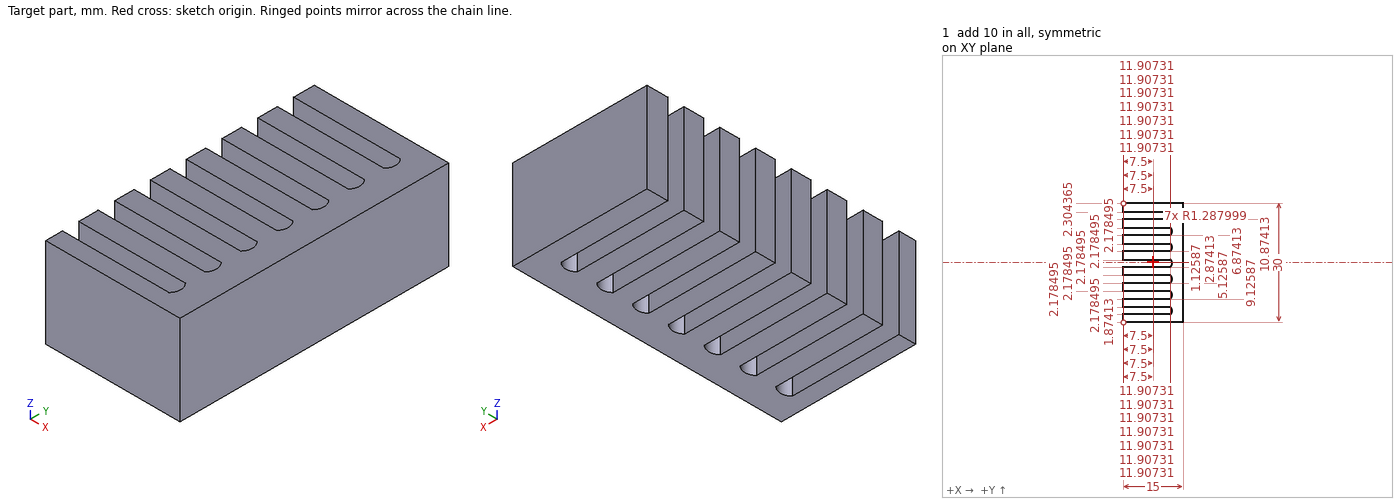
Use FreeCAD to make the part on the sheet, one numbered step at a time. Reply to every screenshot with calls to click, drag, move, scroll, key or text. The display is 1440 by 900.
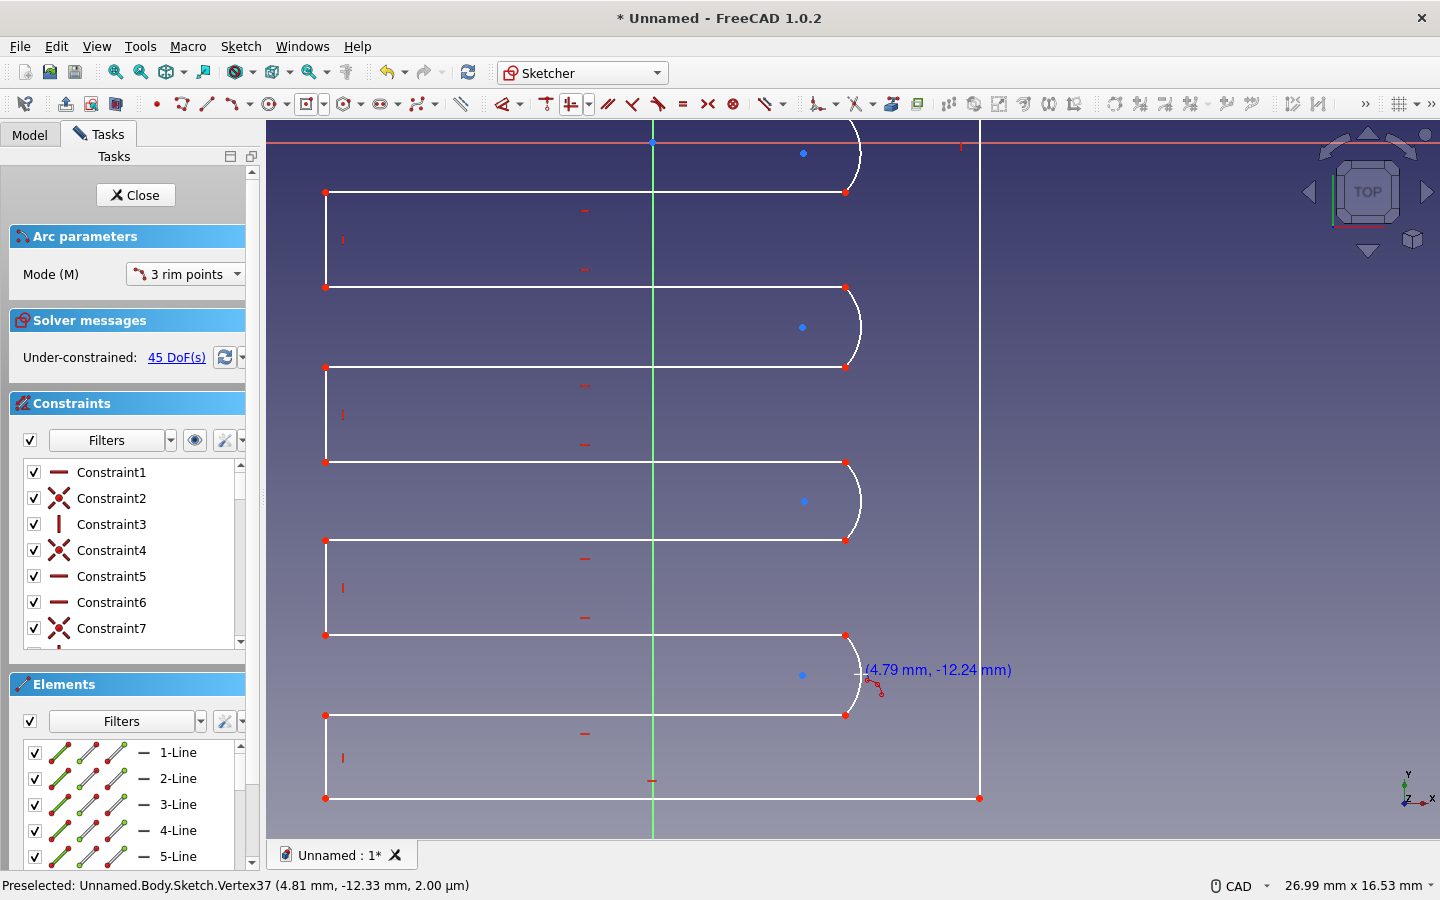
scroll(861, 676, down, 5)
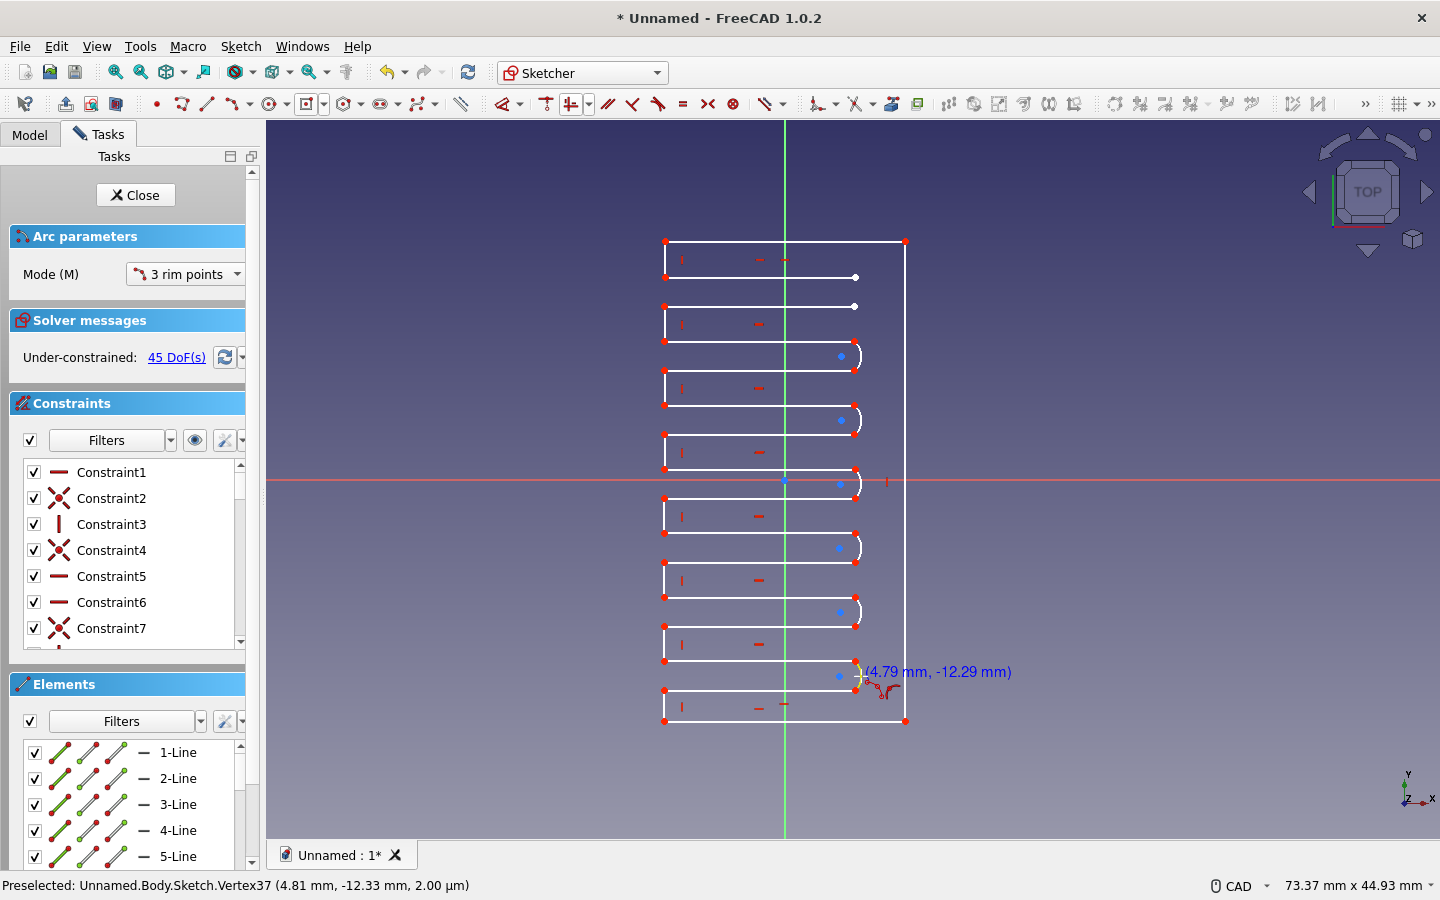
click(855, 278)
click(855, 307)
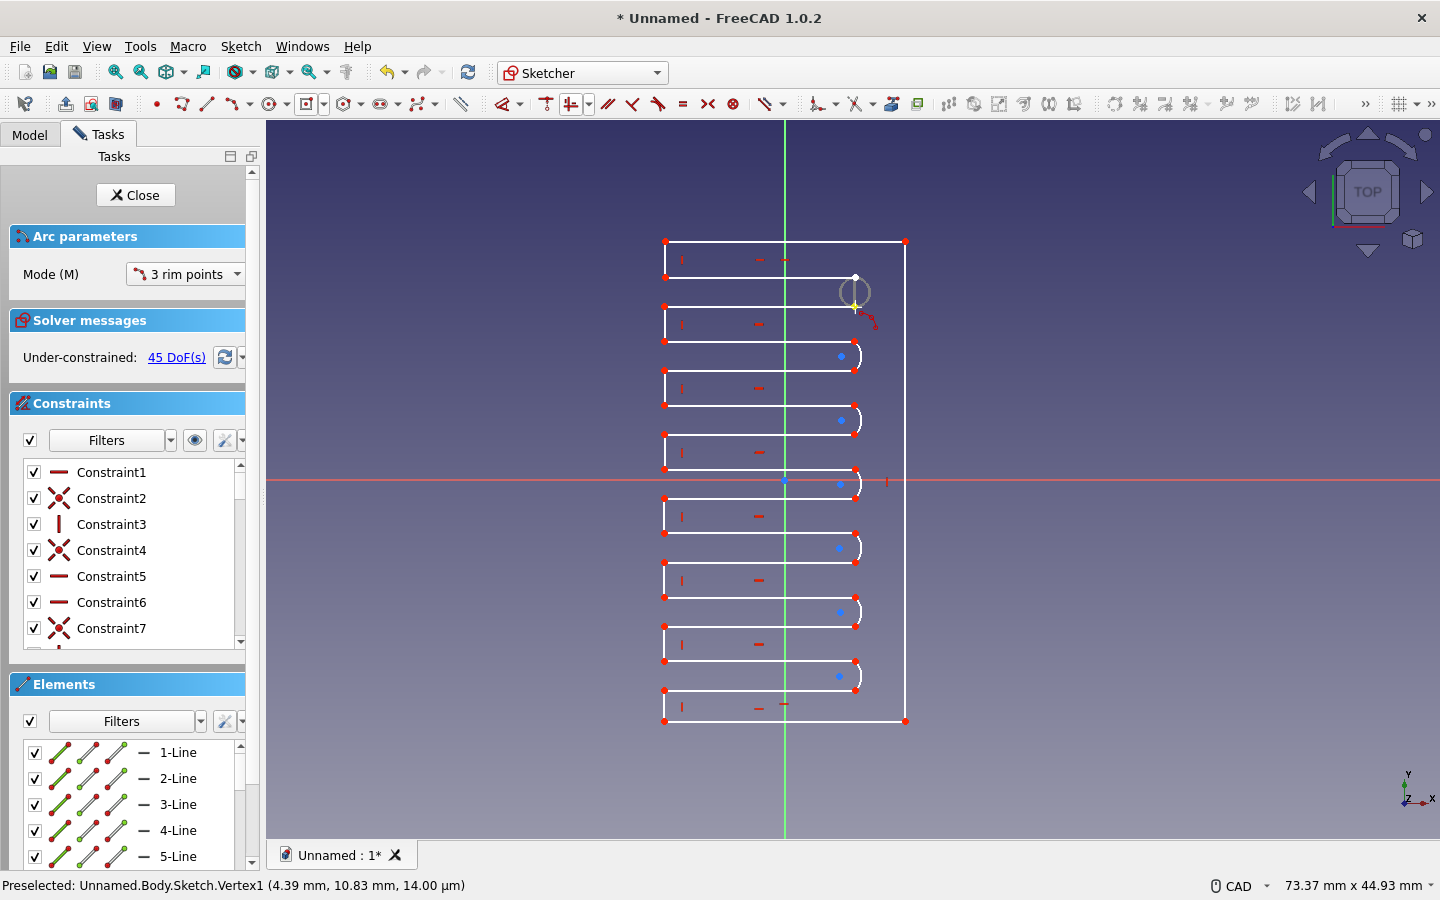
scroll(861, 292, up, 5)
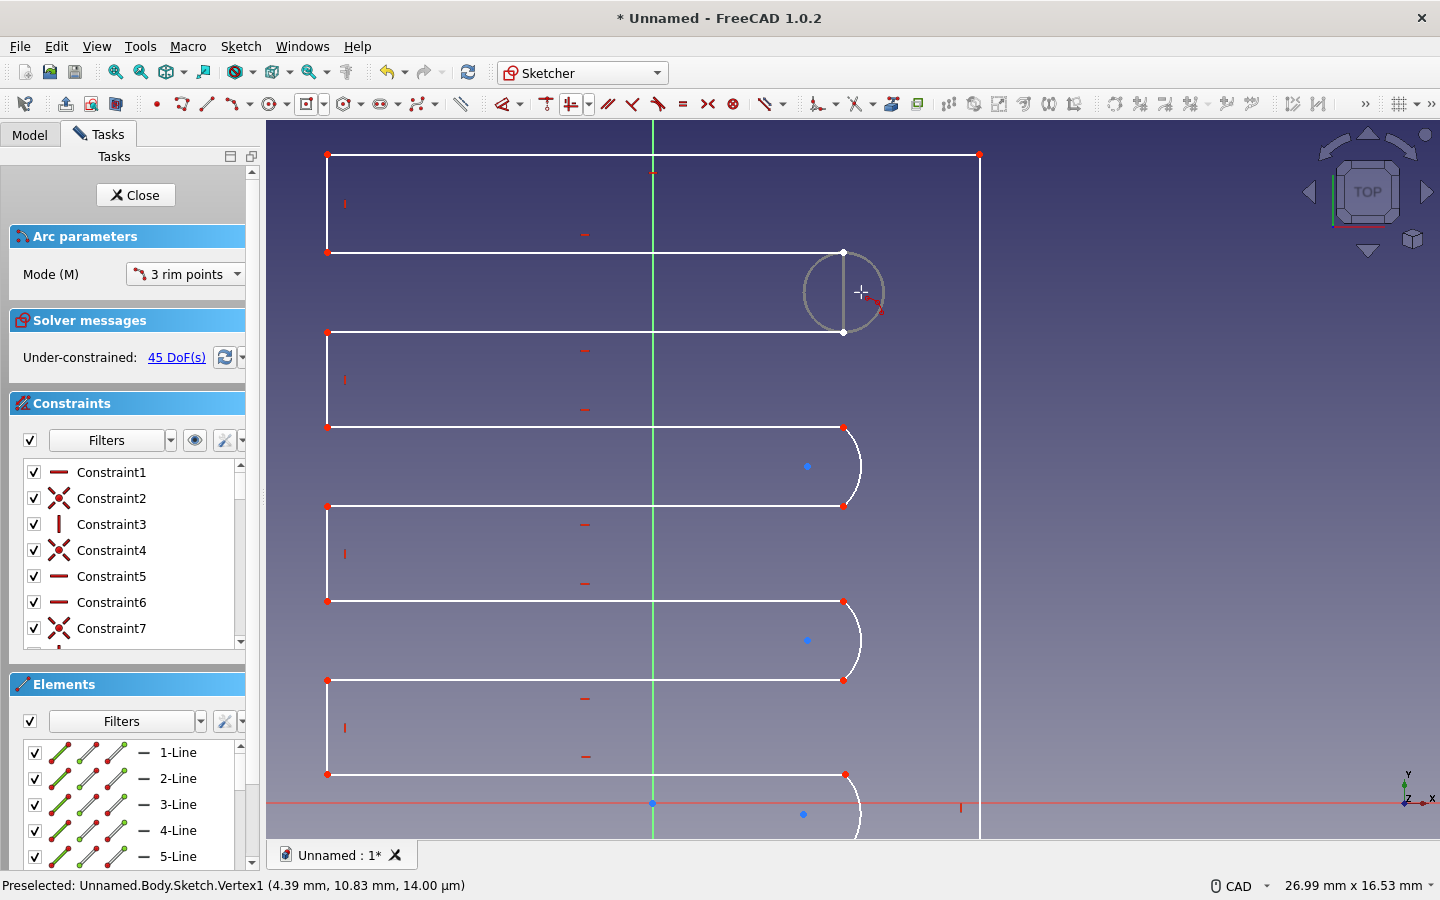
click(861, 291)
key(Escape)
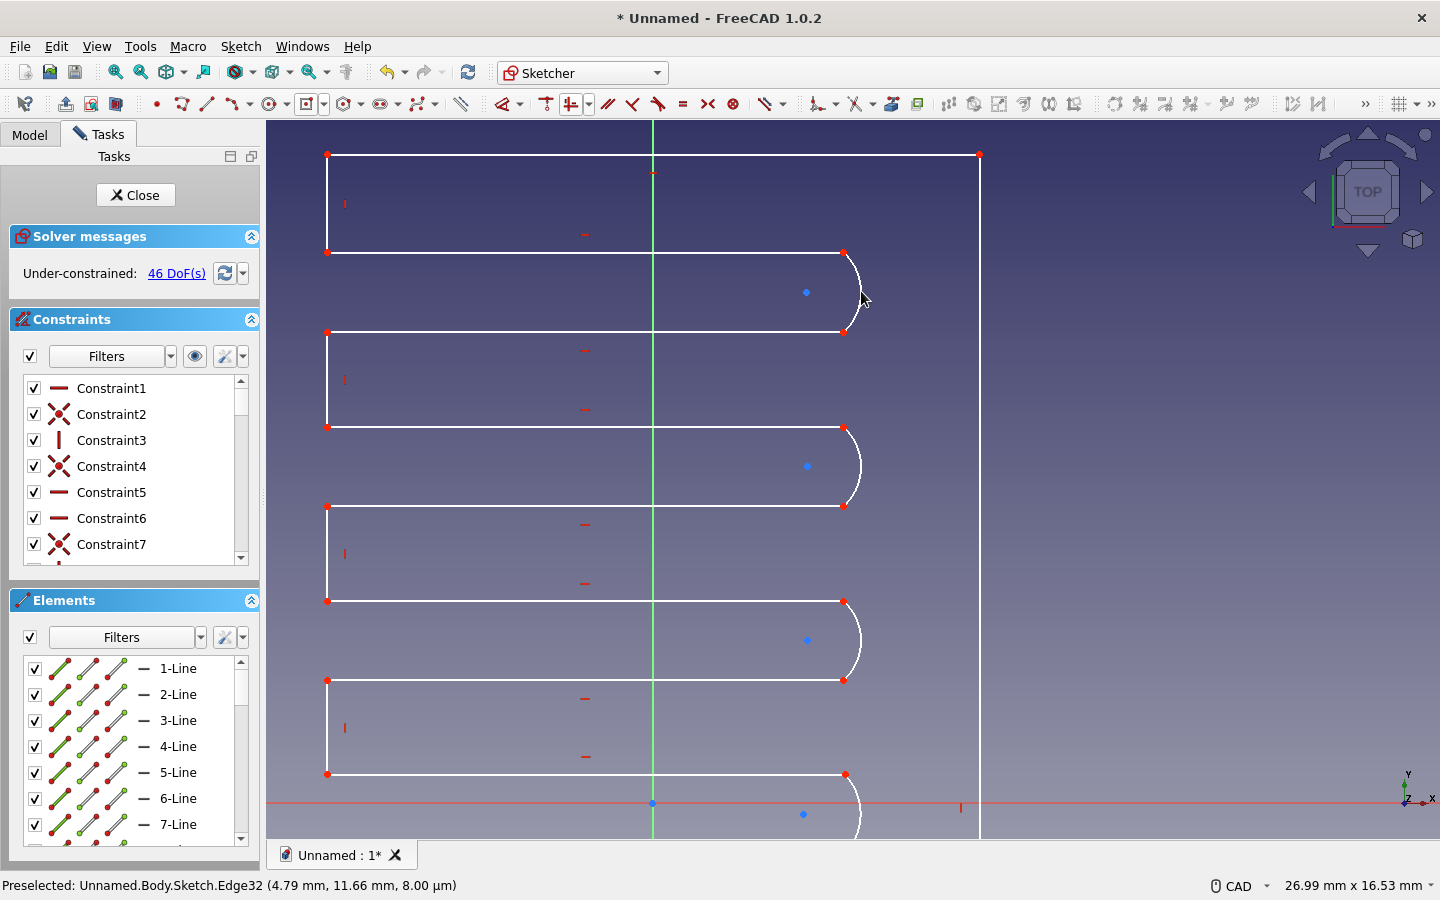
click(858, 484)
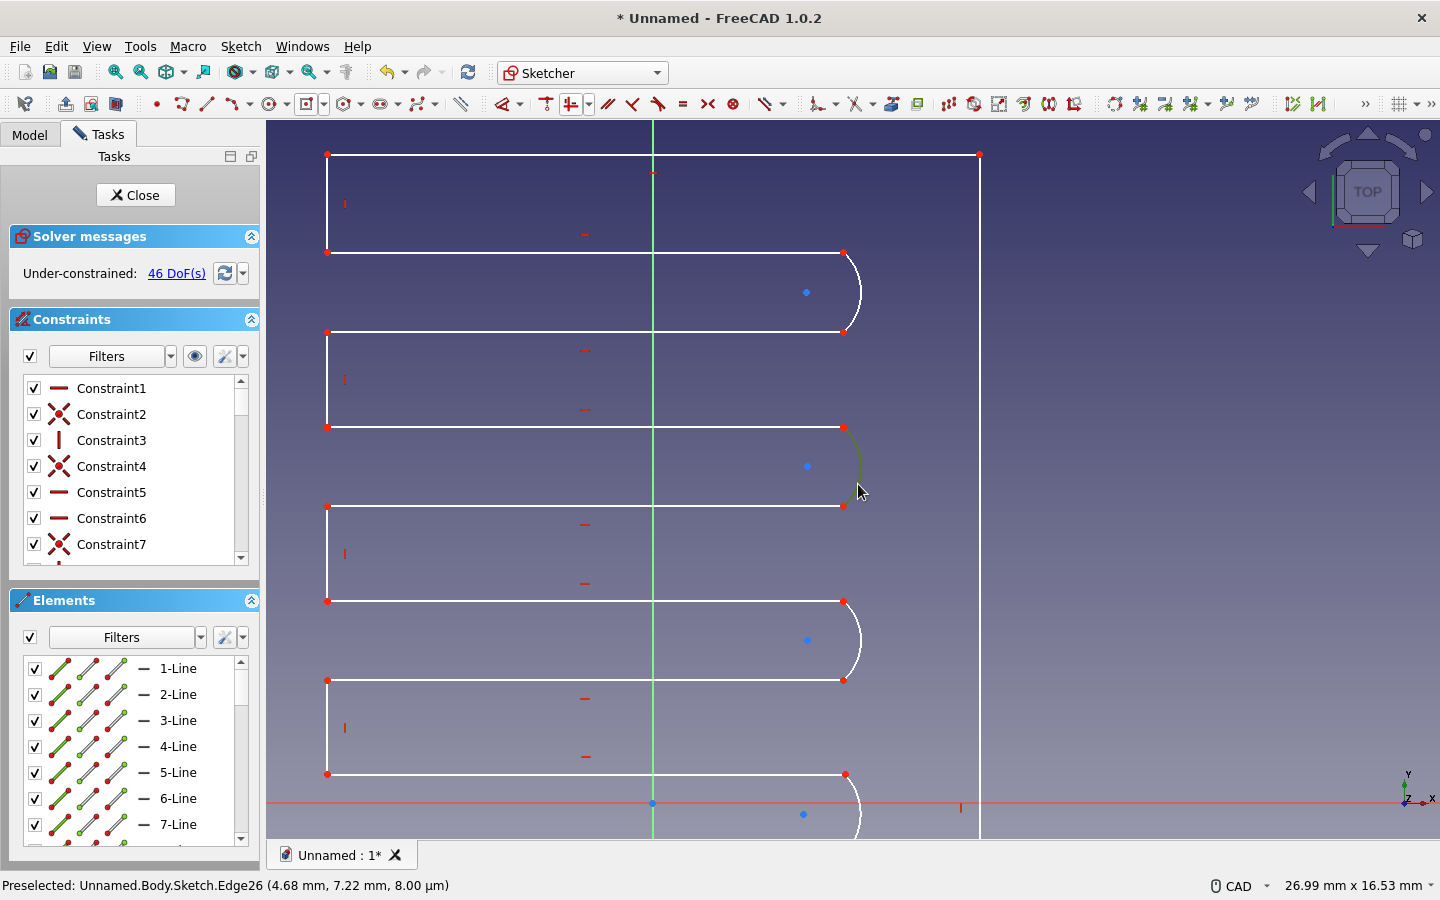
click(858, 658)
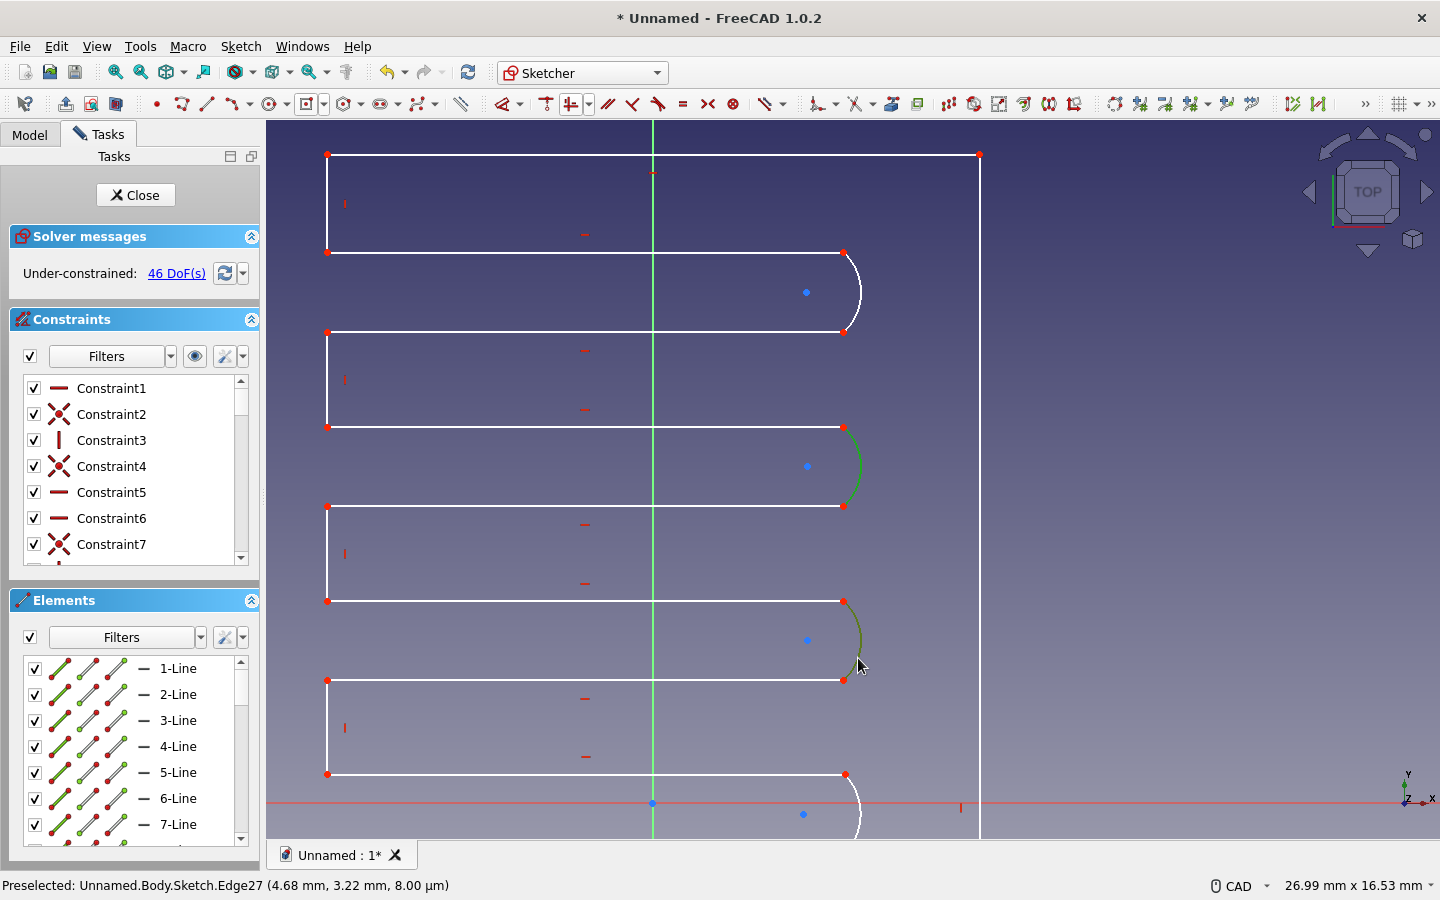
click(855, 789)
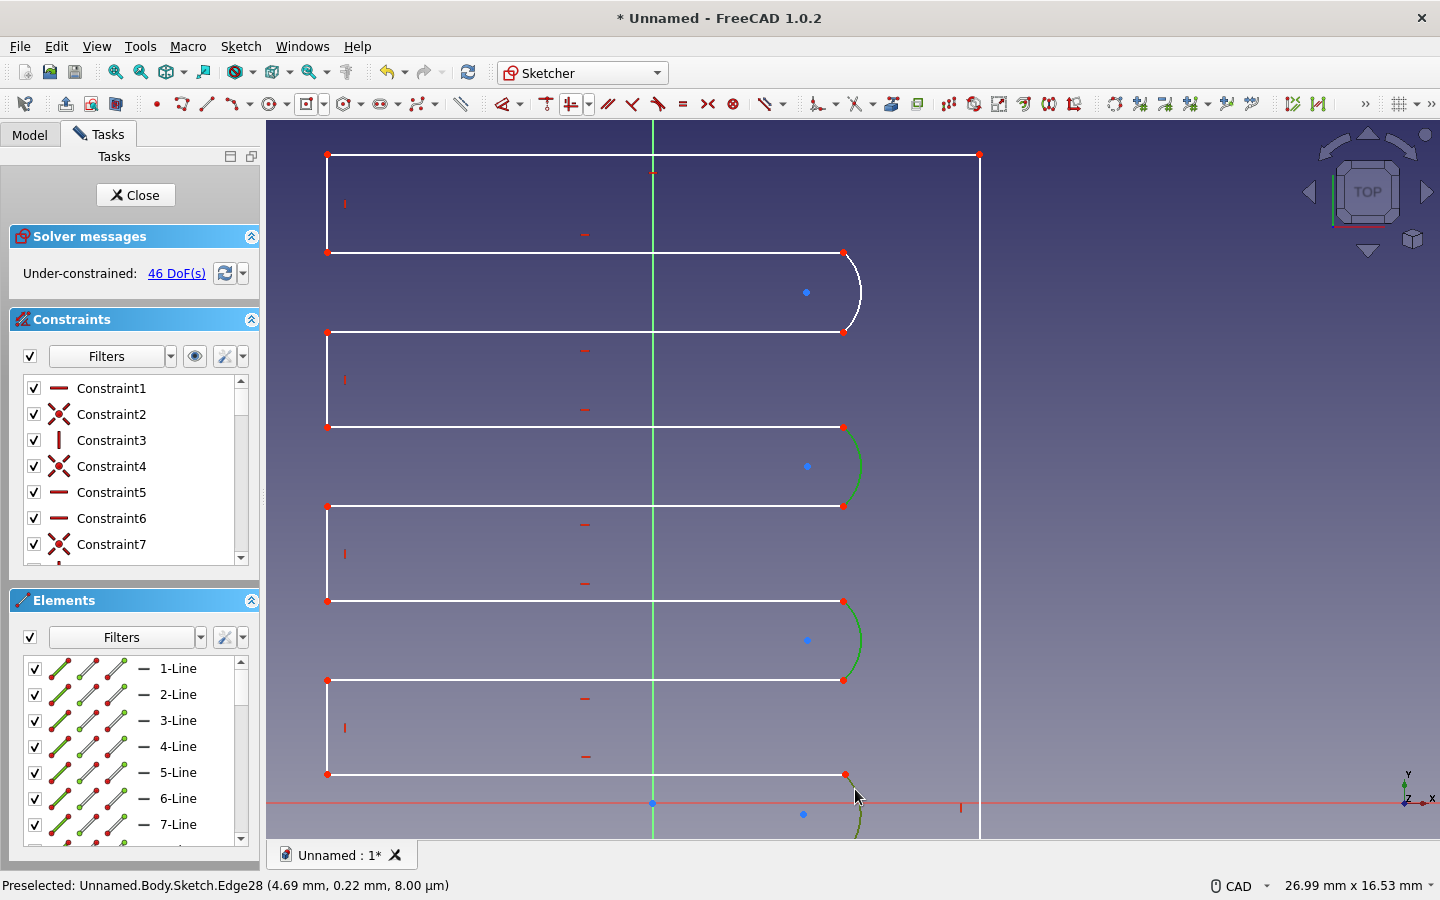
scroll(861, 291, down, 5)